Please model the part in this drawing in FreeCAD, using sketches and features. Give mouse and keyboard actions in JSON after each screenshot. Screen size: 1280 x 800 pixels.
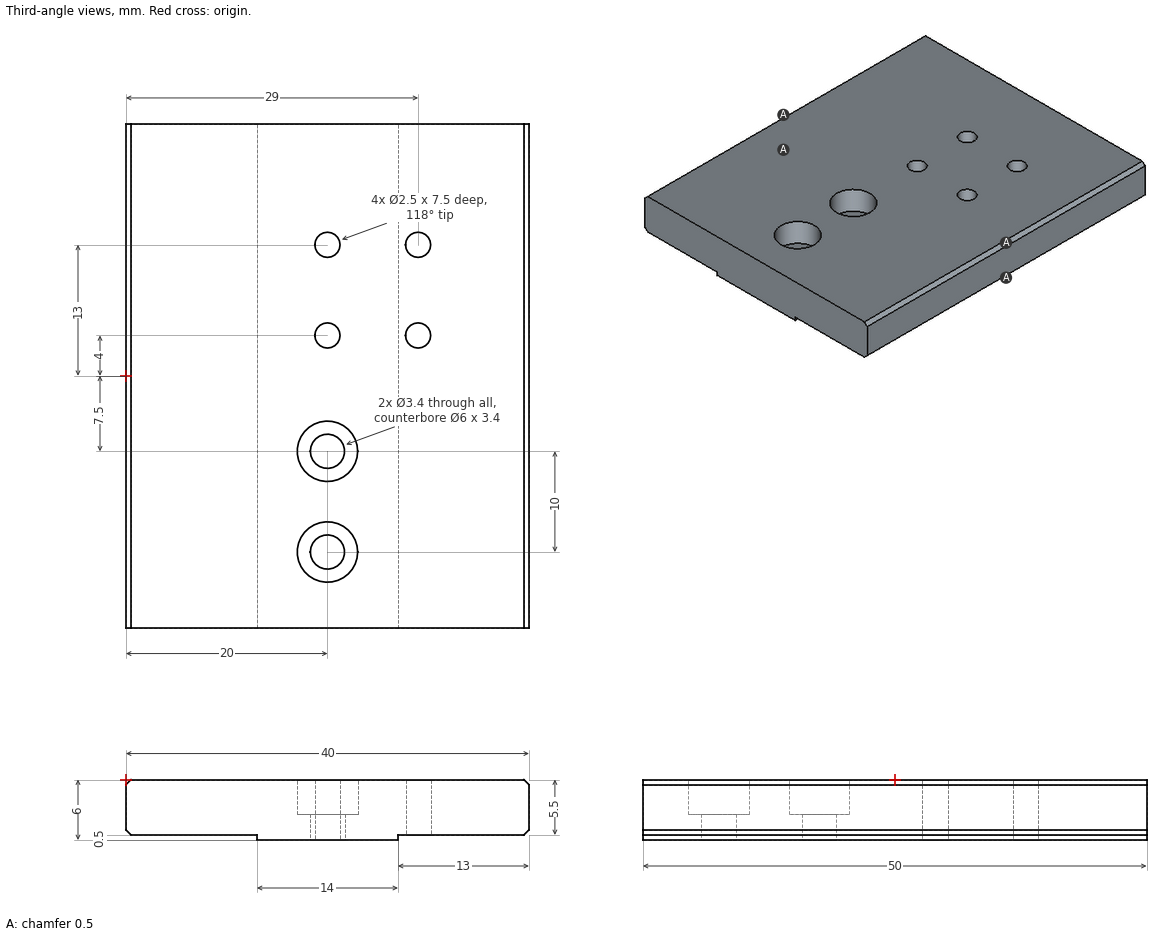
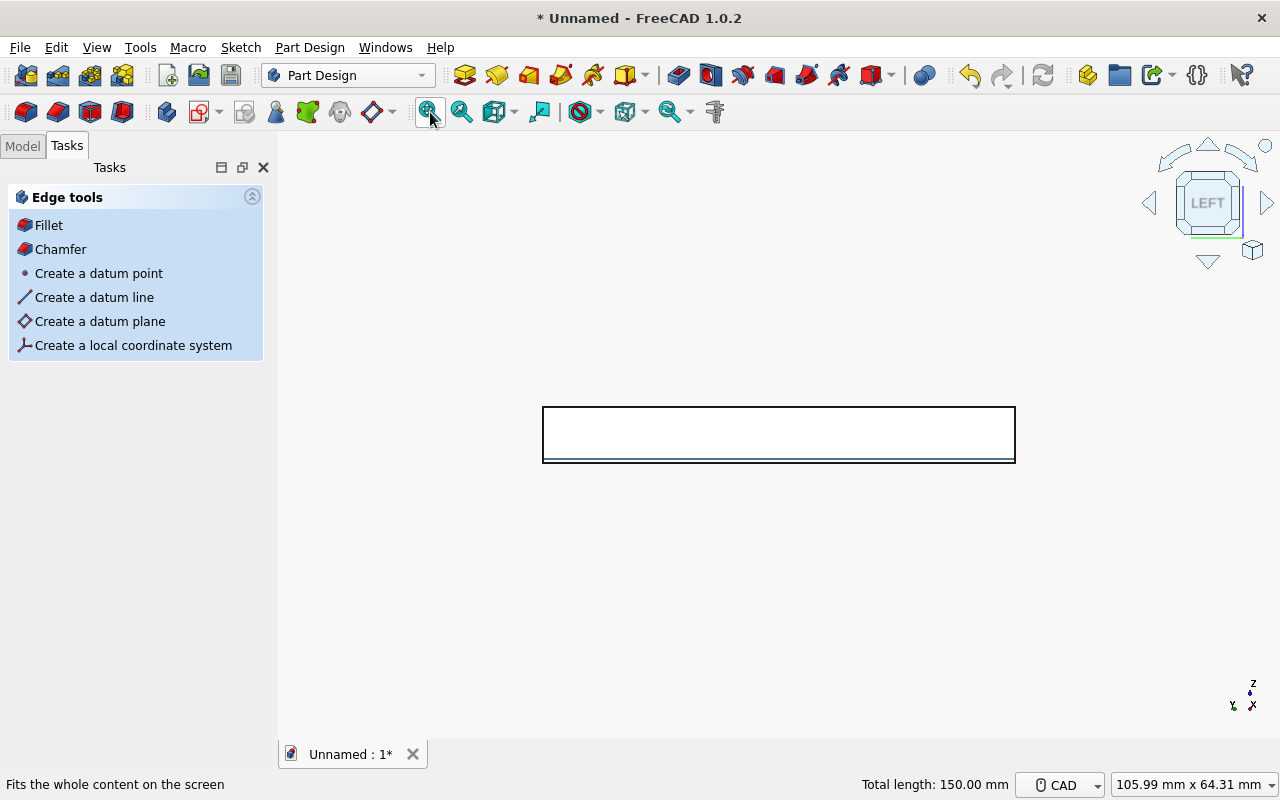
{"action": "key", "text": "v 3"}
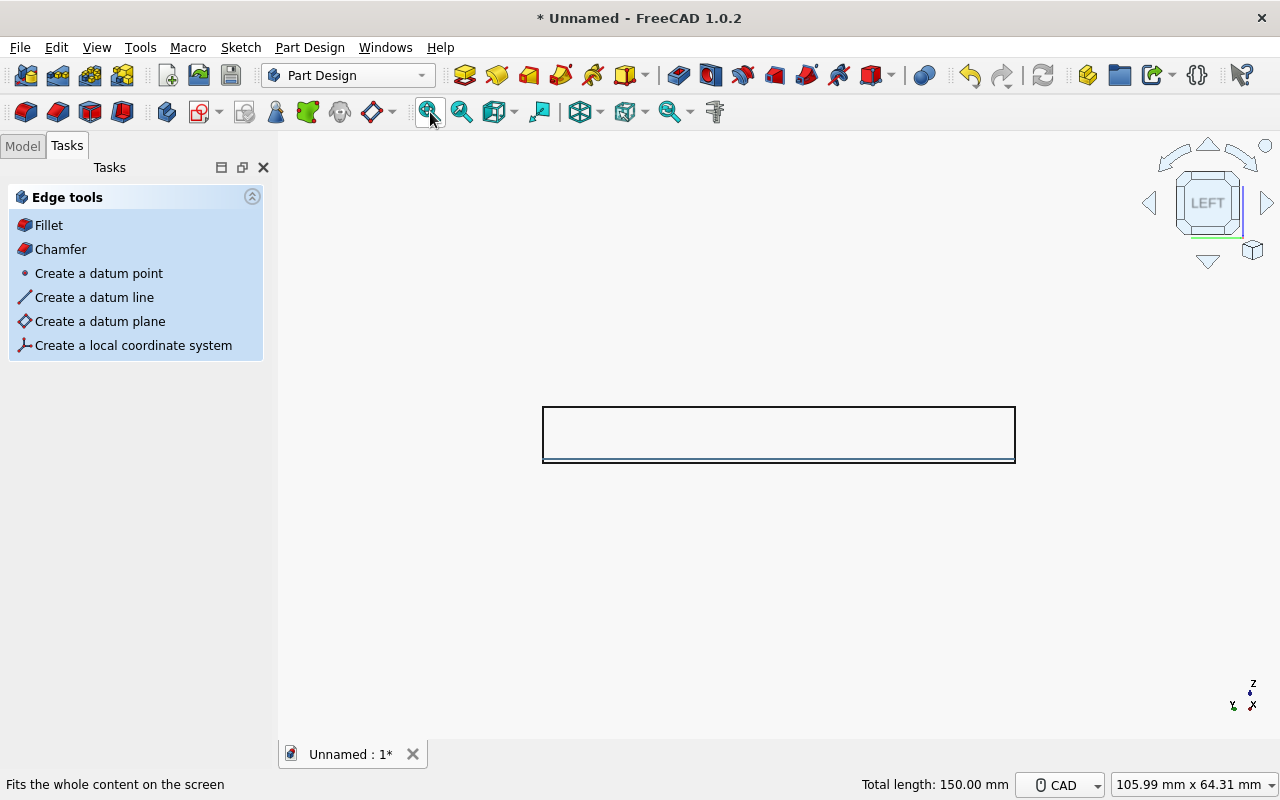
{"action": "key", "text": "0"}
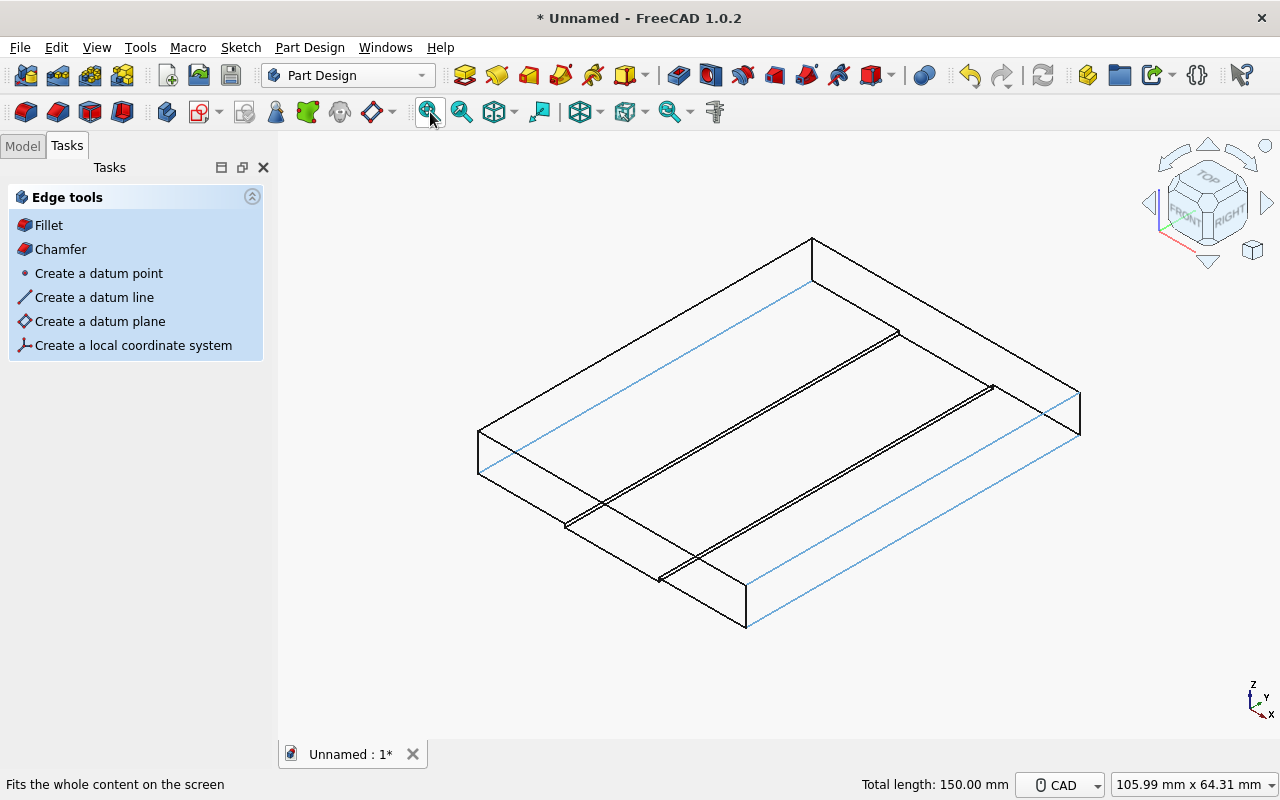
{"action": "left_click", "coordinate": [645, 334], "text": "ctrl"}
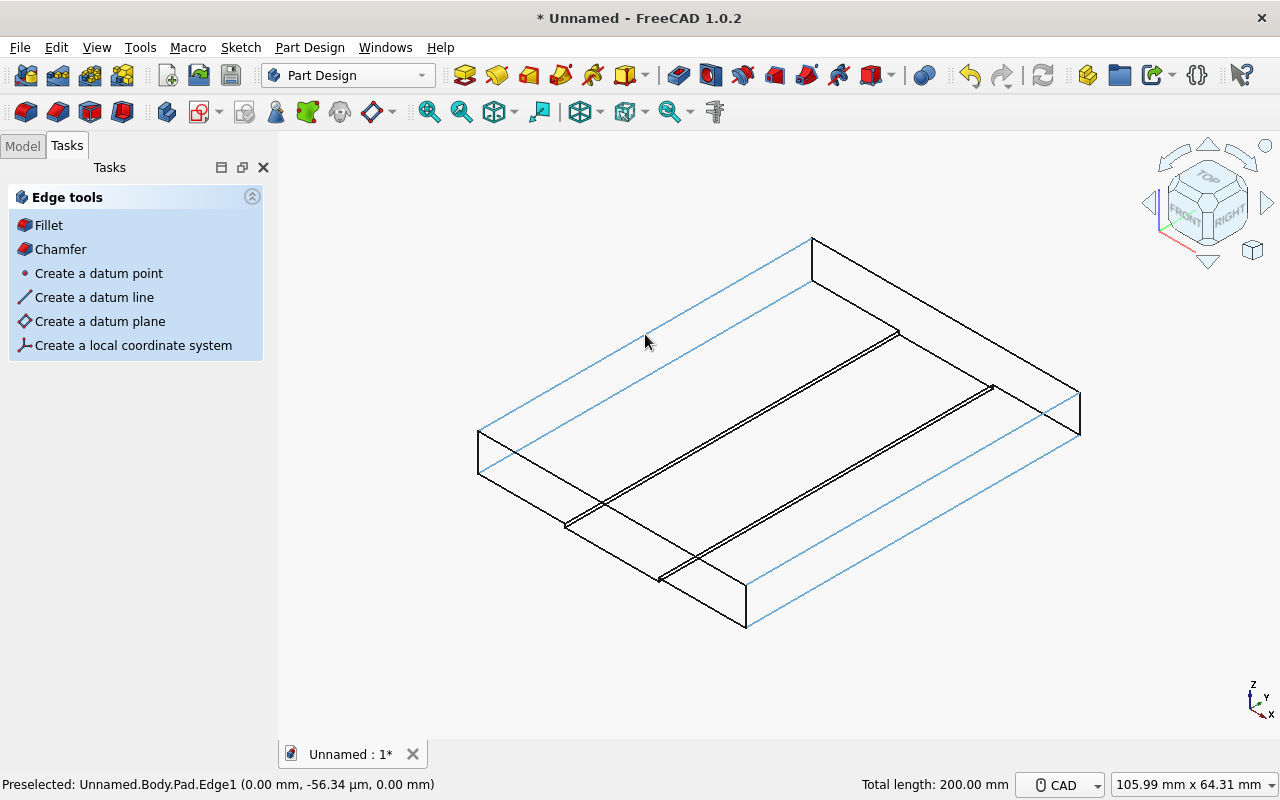
{"action": "key", "text": "v 1"}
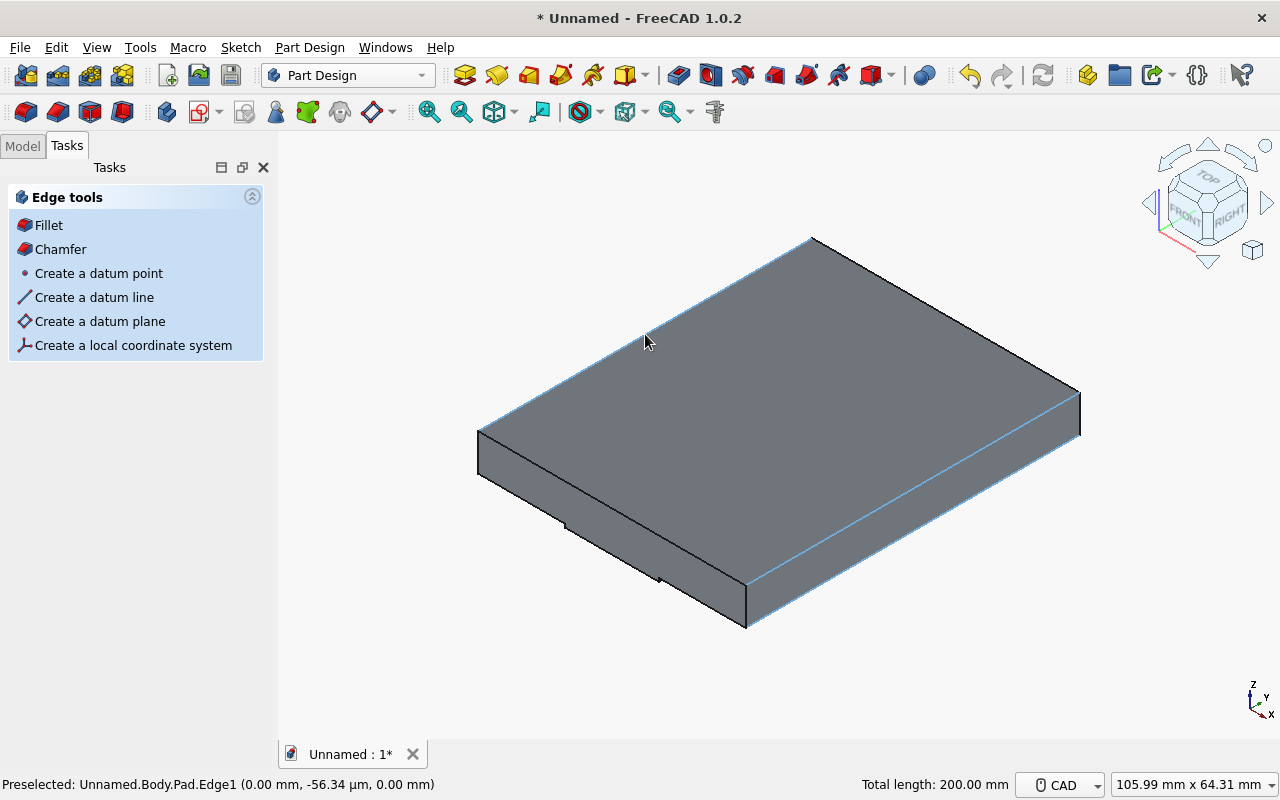
{"action": "left_click", "coordinate": [58, 112]}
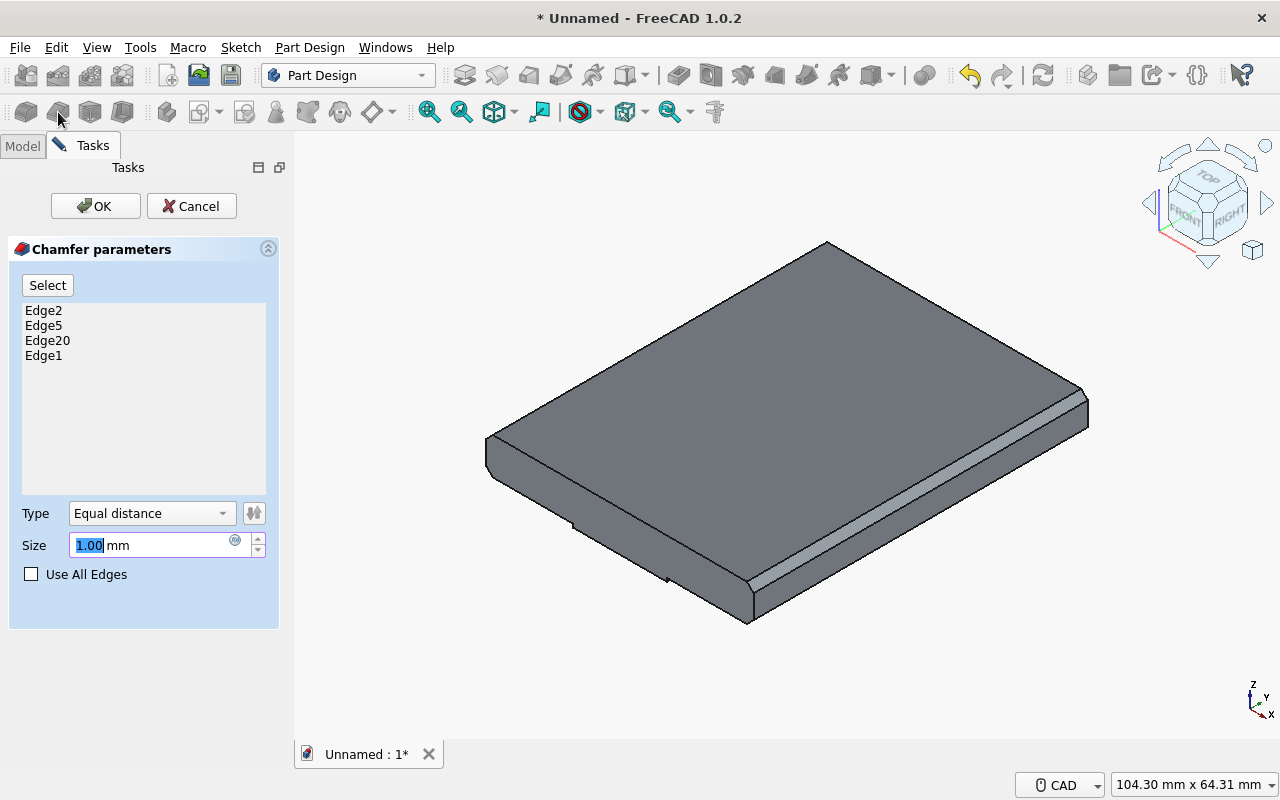
{"action": "type", "text": "0.5"}
{"action": "key", "text": "Tab"}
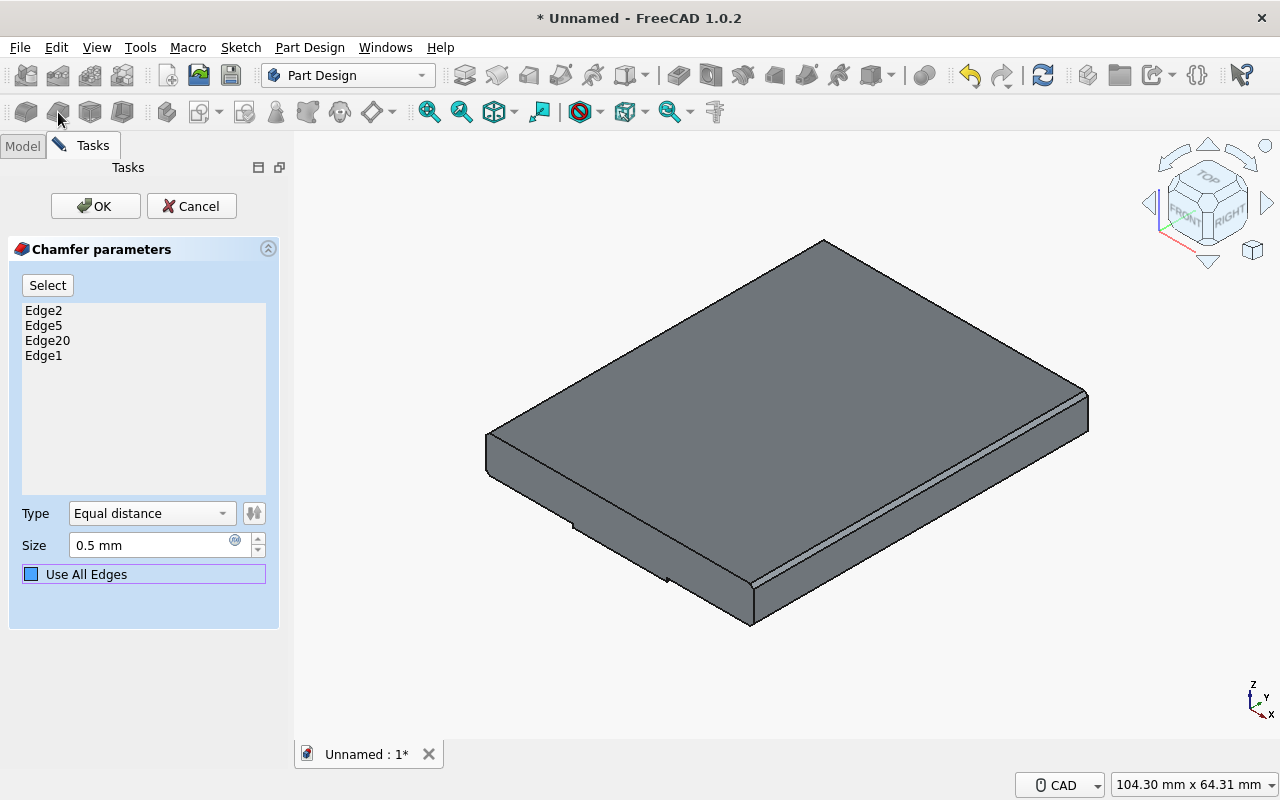
{"action": "left_click", "coordinate": [96, 206]}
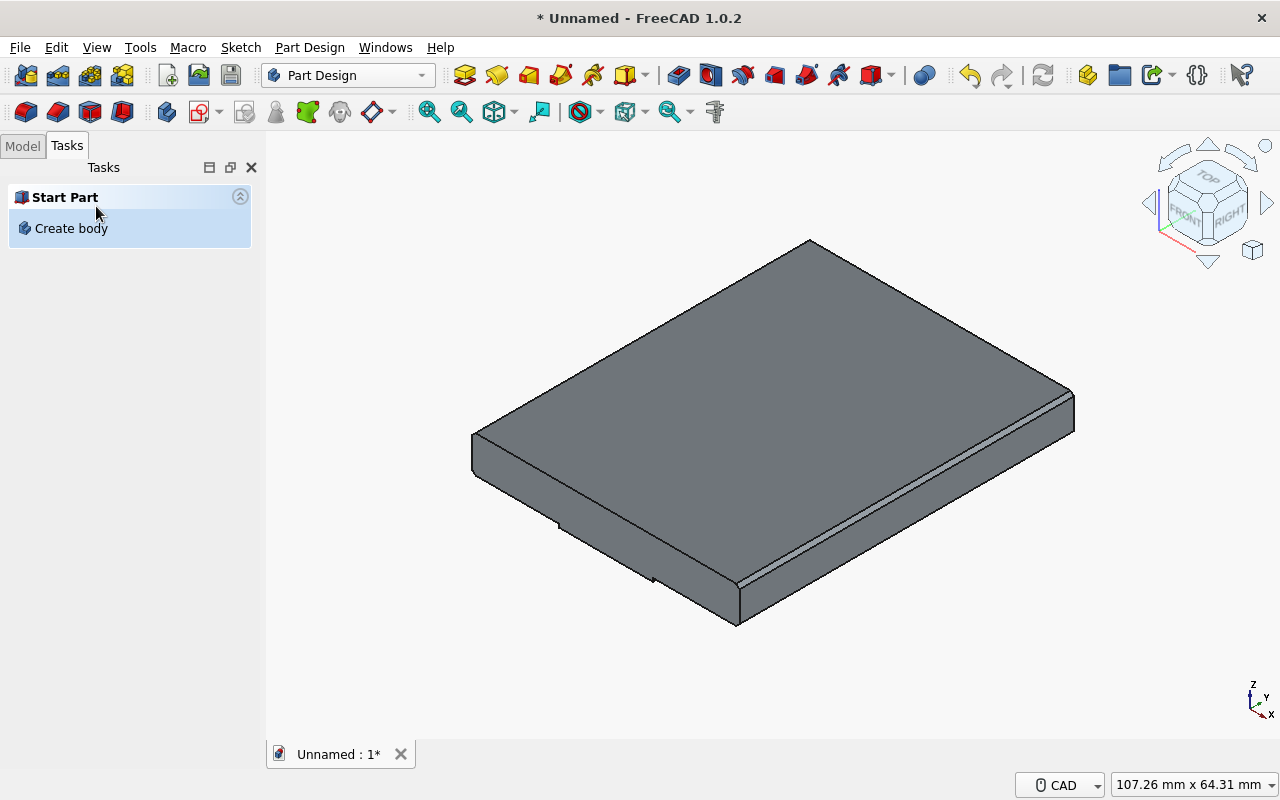
{"action": "left_click", "coordinate": [200, 112]}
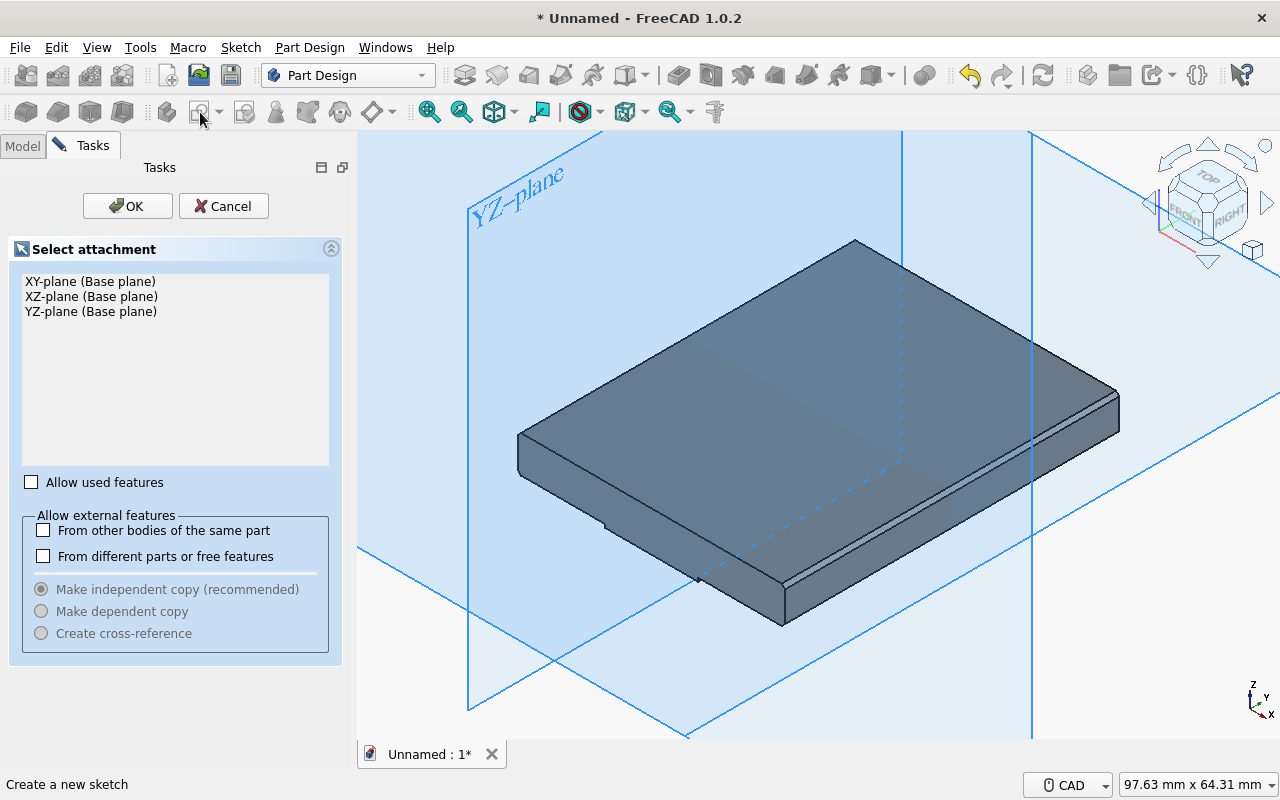
{"action": "left_click", "coordinate": [82, 282]}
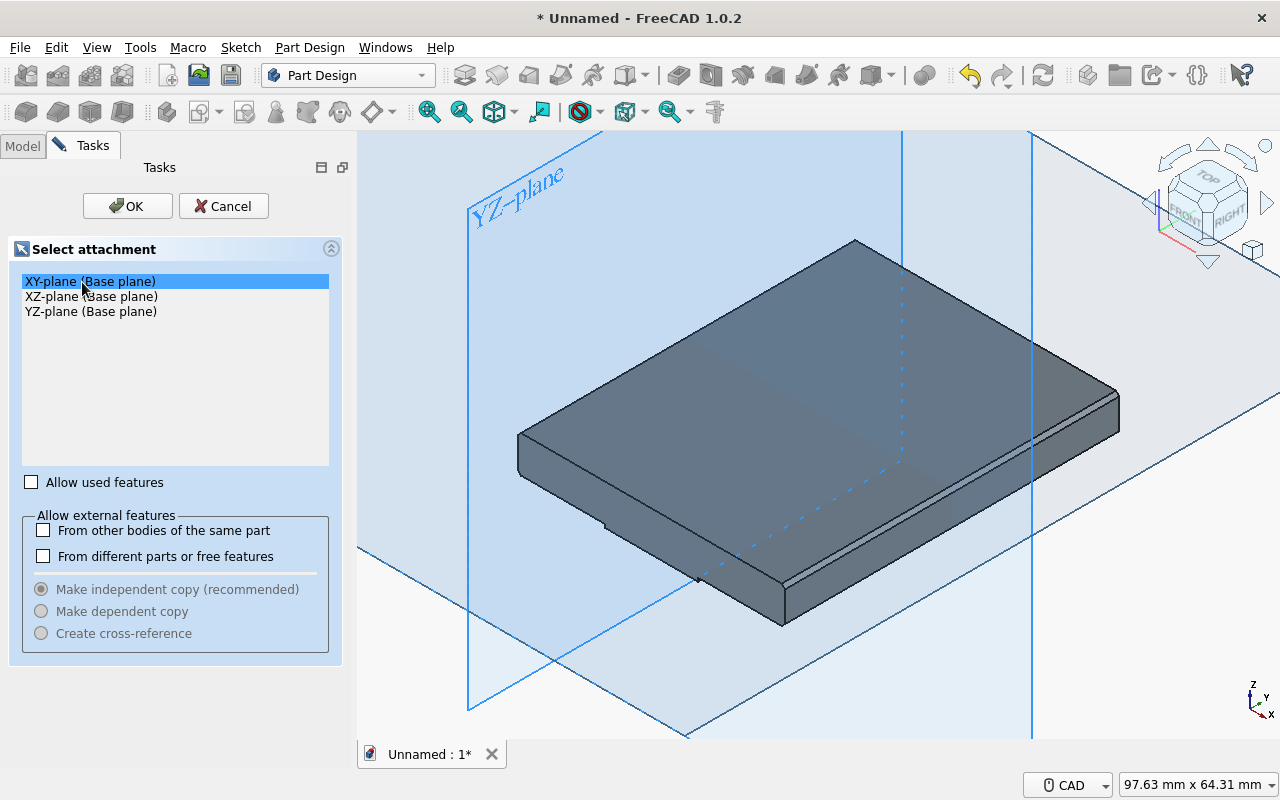
{"action": "left_click", "coordinate": [128, 206]}